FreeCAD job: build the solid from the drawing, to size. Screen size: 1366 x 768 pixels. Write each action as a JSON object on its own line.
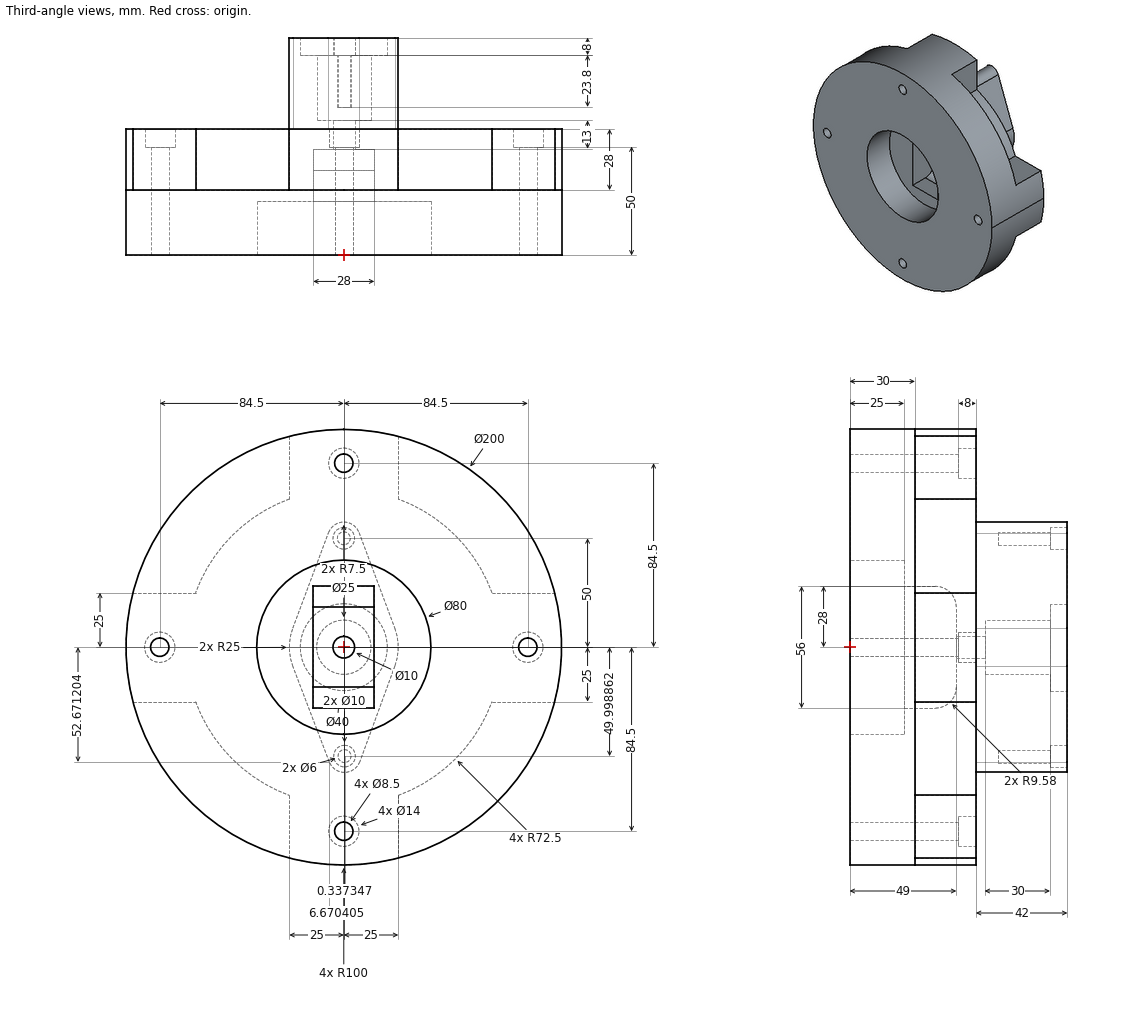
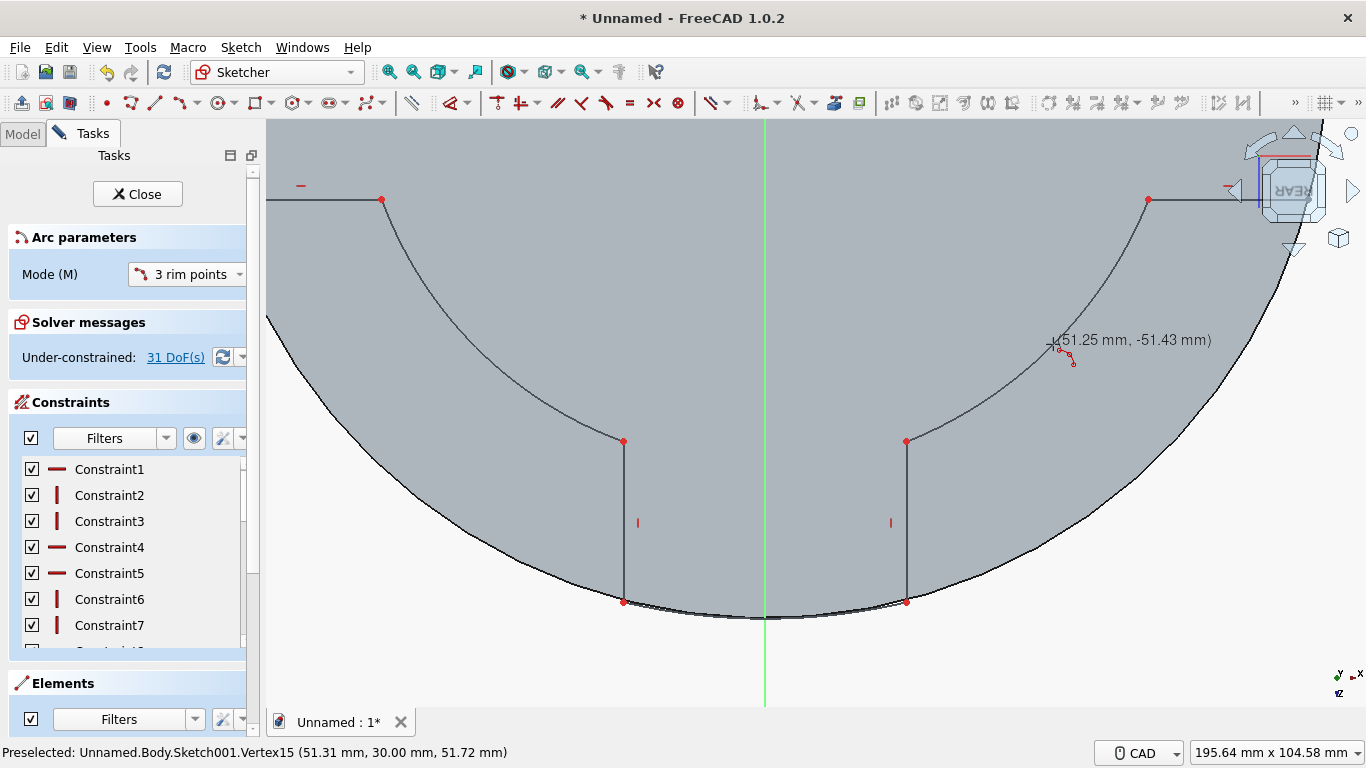
{"action": "scroll", "coordinate": [737, 621], "scroll_direction": "down", "scroll_amount": 5}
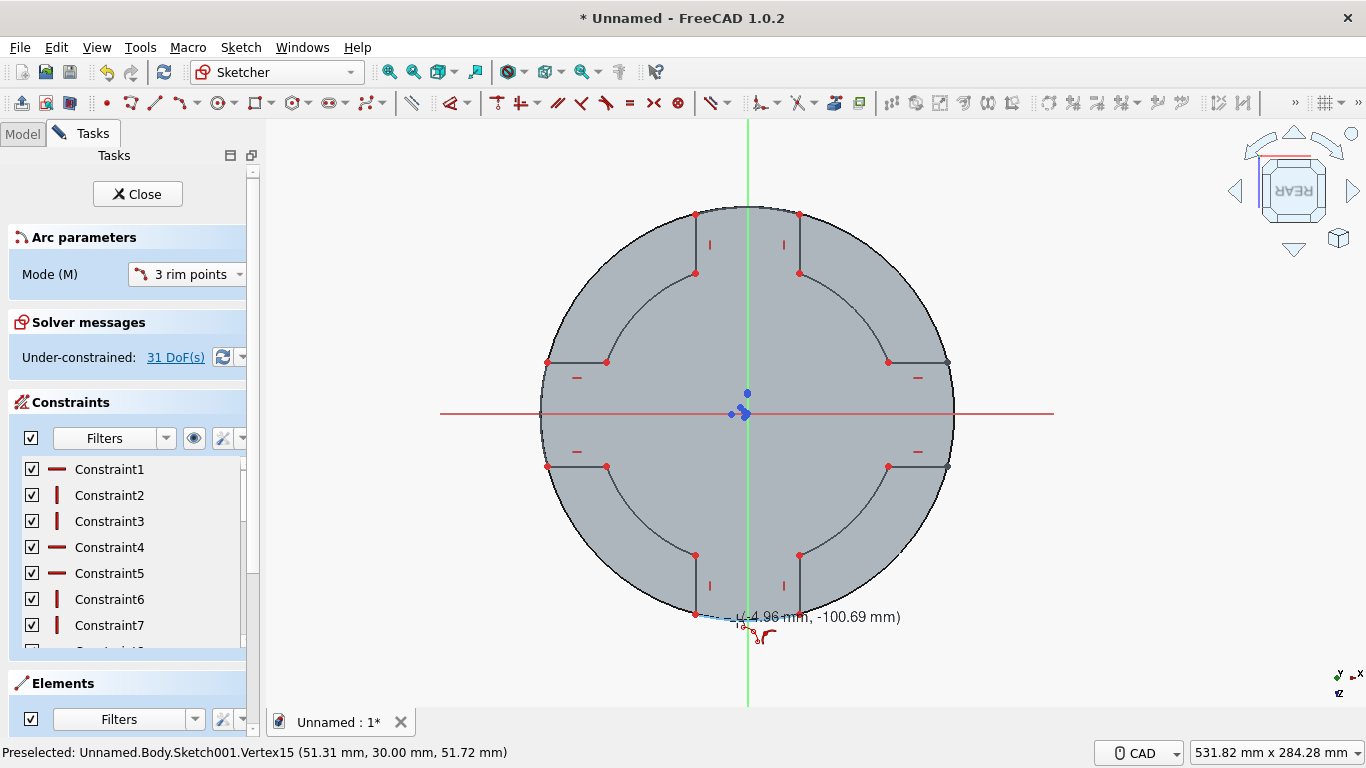
{"action": "left_click", "coordinate": [948, 467]}
{"action": "left_click", "coordinate": [948, 363]}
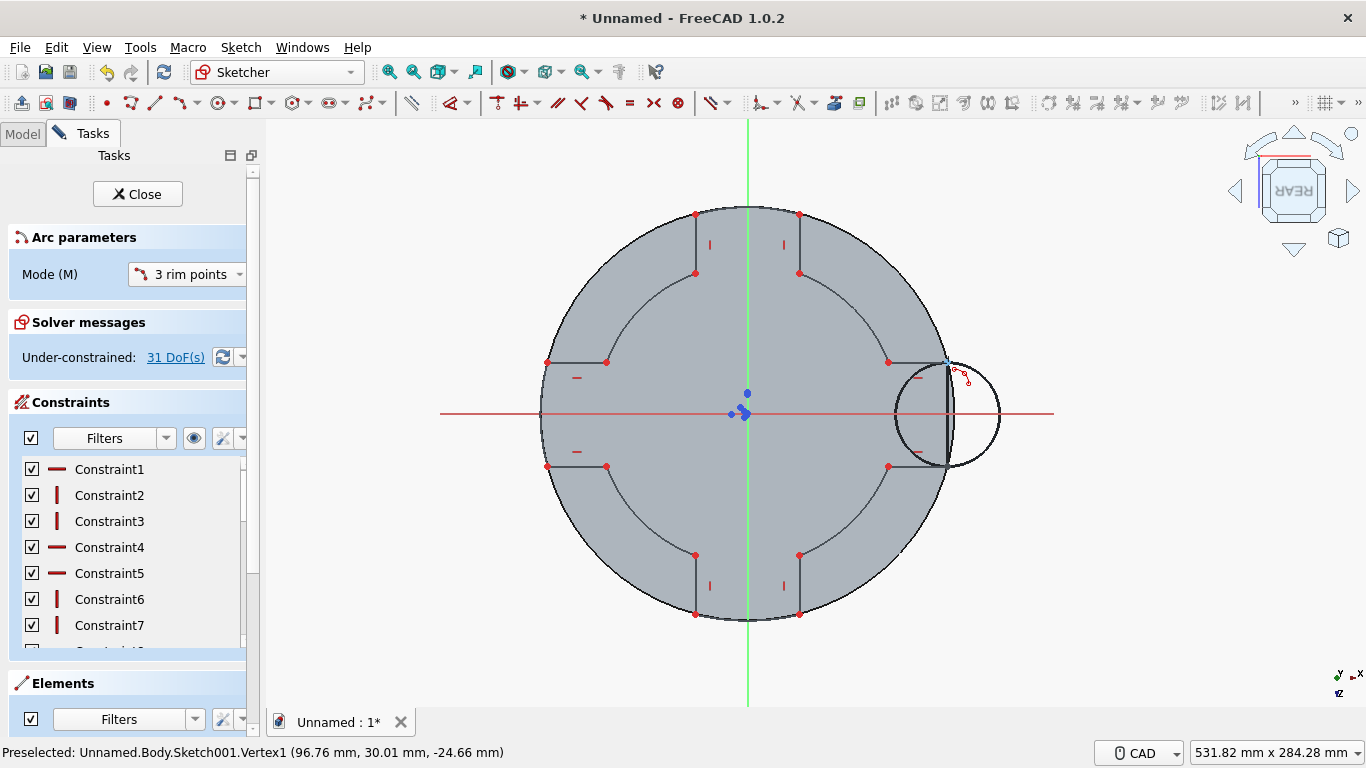
{"action": "scroll", "coordinate": [954, 424], "scroll_direction": "up", "scroll_amount": 5}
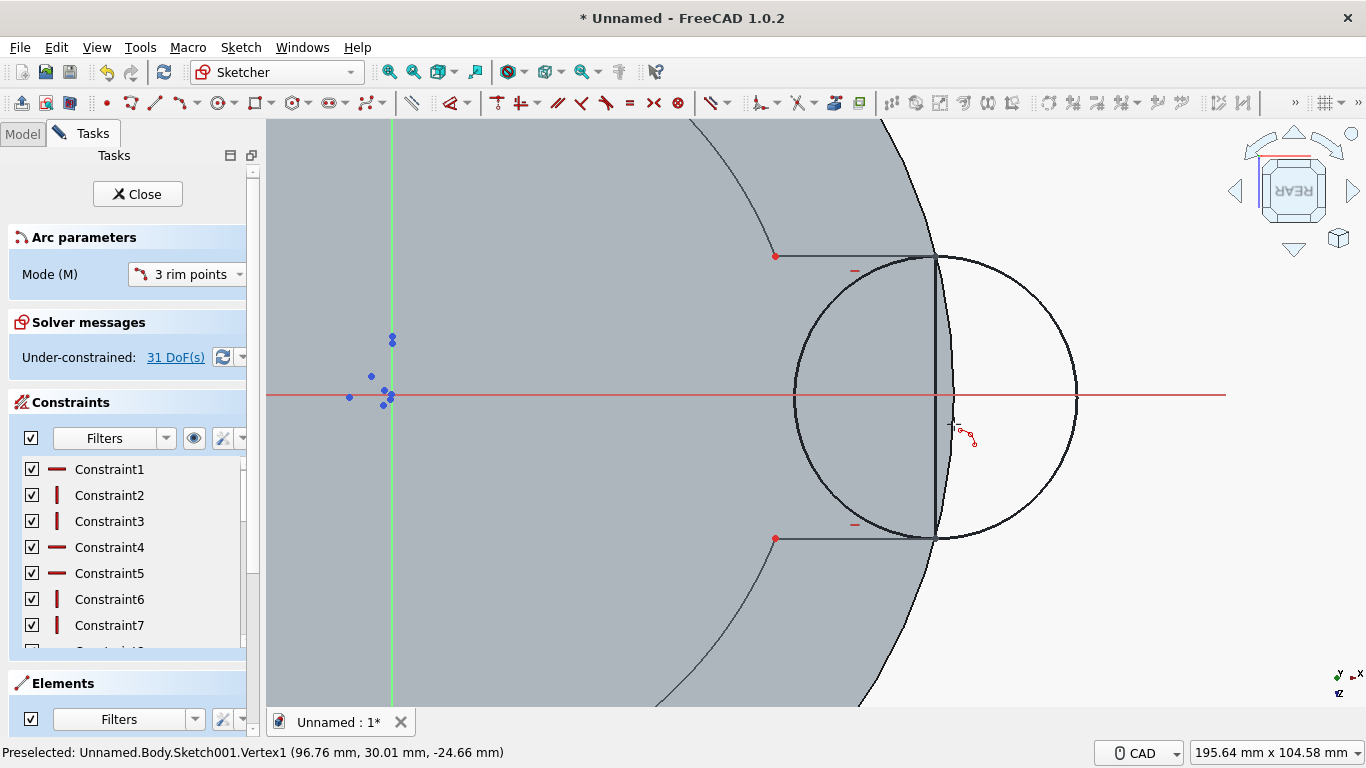
{"action": "left_click", "coordinate": [953, 423]}
{"action": "key", "text": "Escape"}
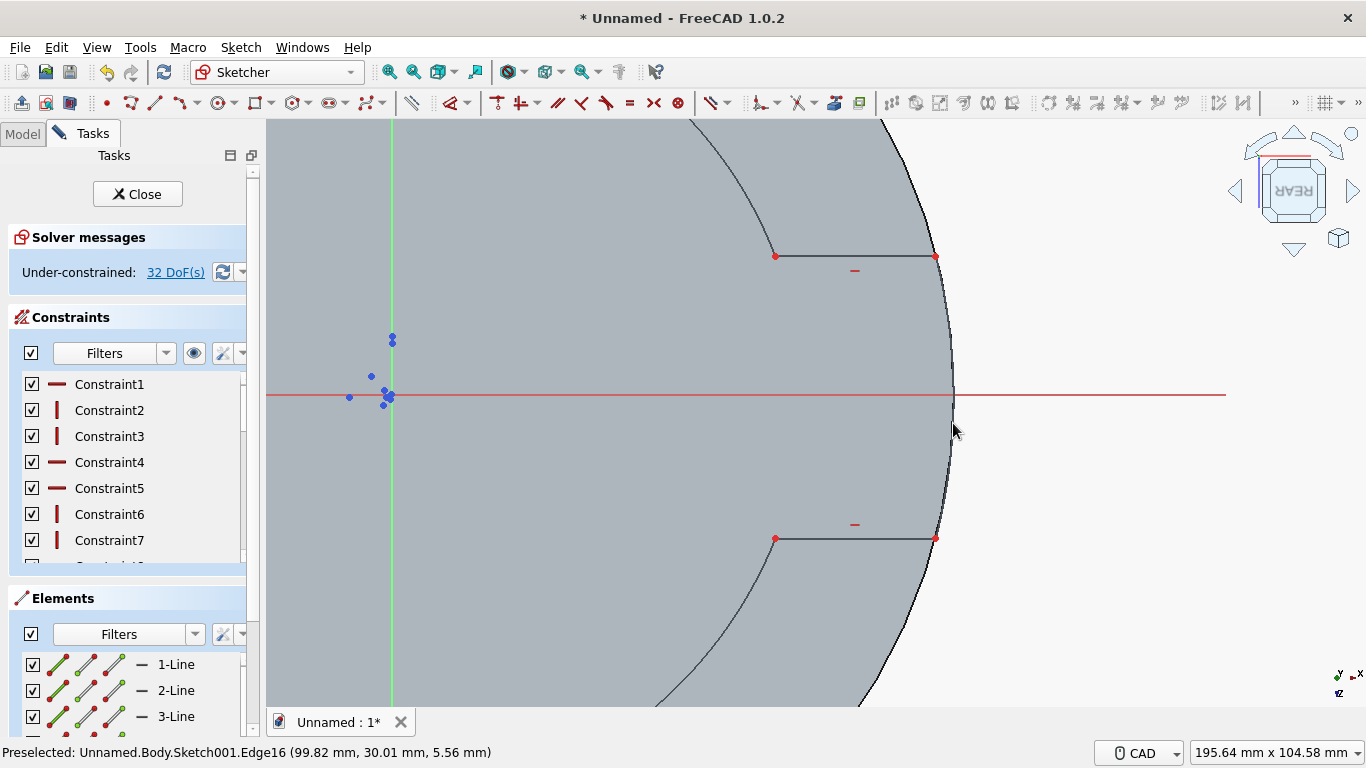
{"action": "left_click", "coordinate": [726, 163]}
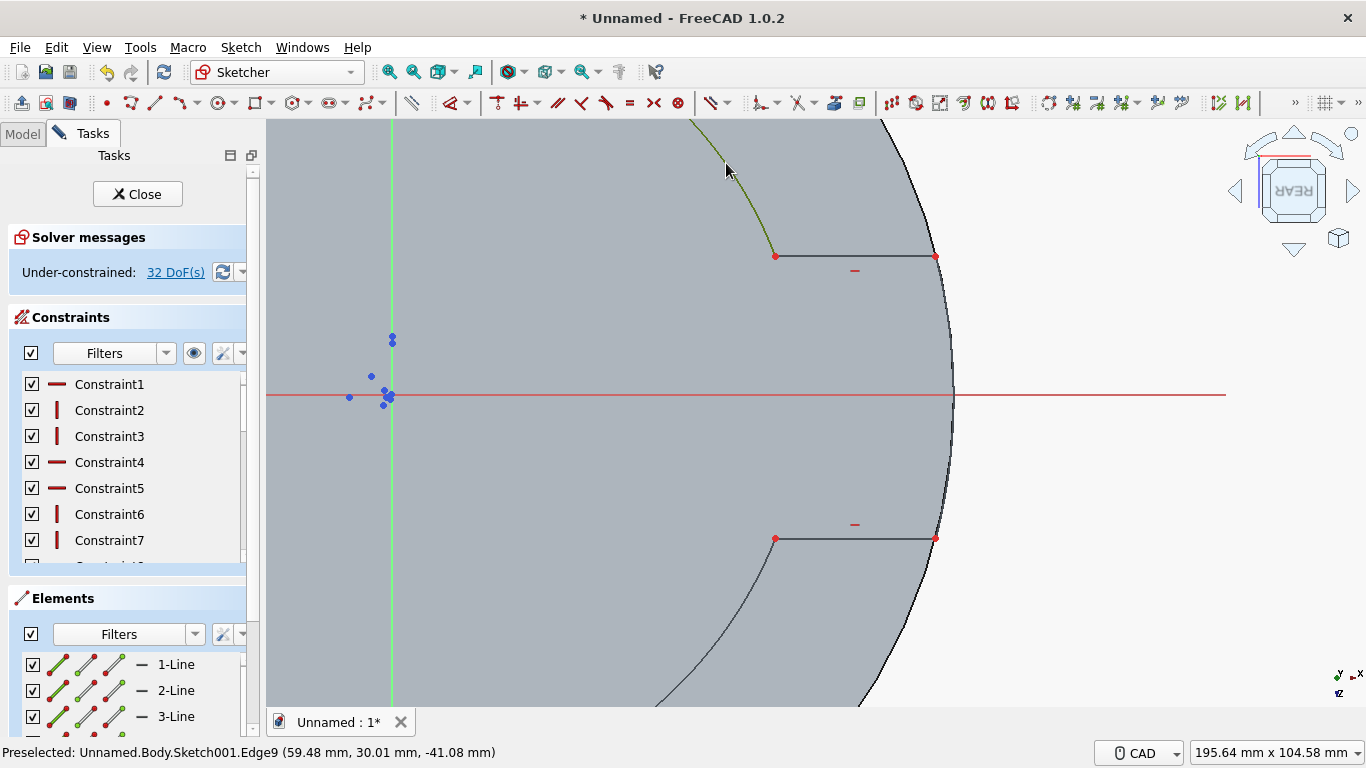
{"action": "scroll", "coordinate": [955, 424], "scroll_direction": "down", "scroll_amount": 5}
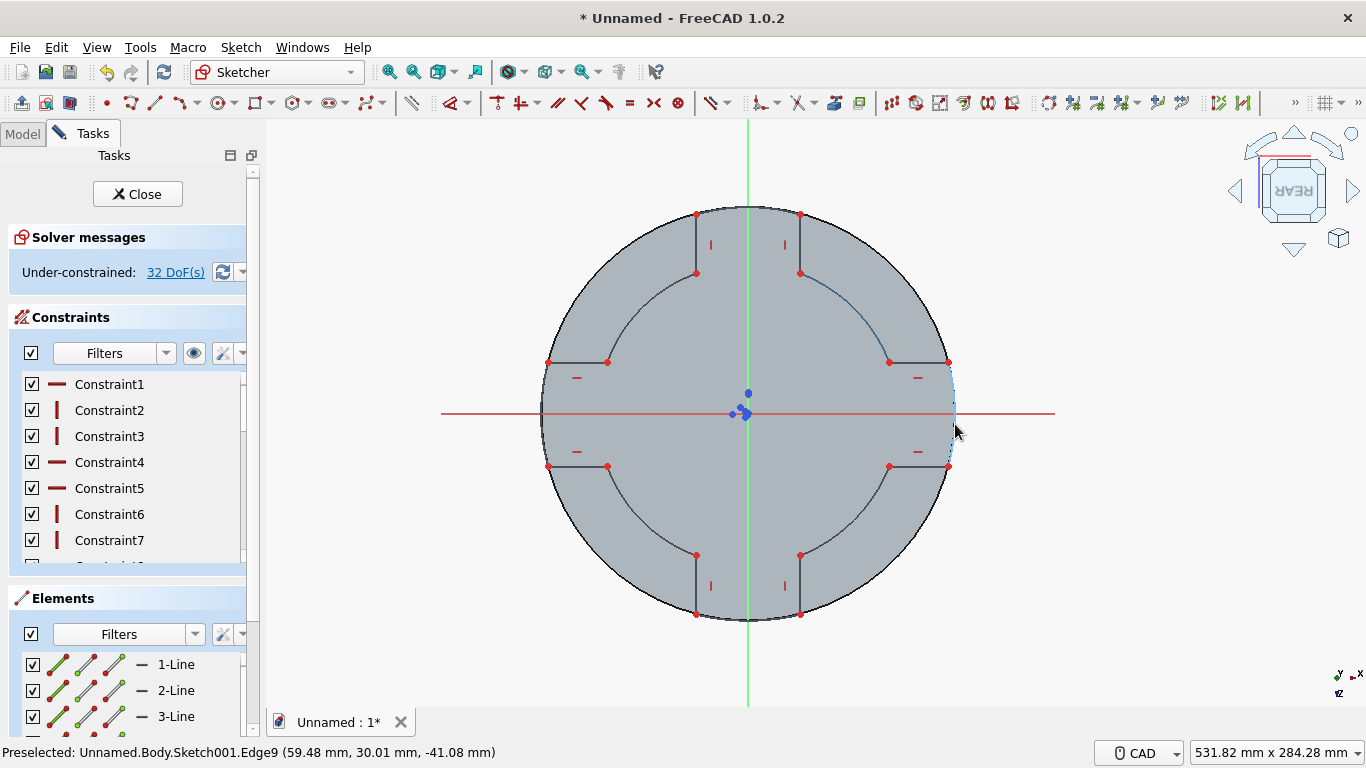
{"action": "left_click", "coordinate": [769, 208]}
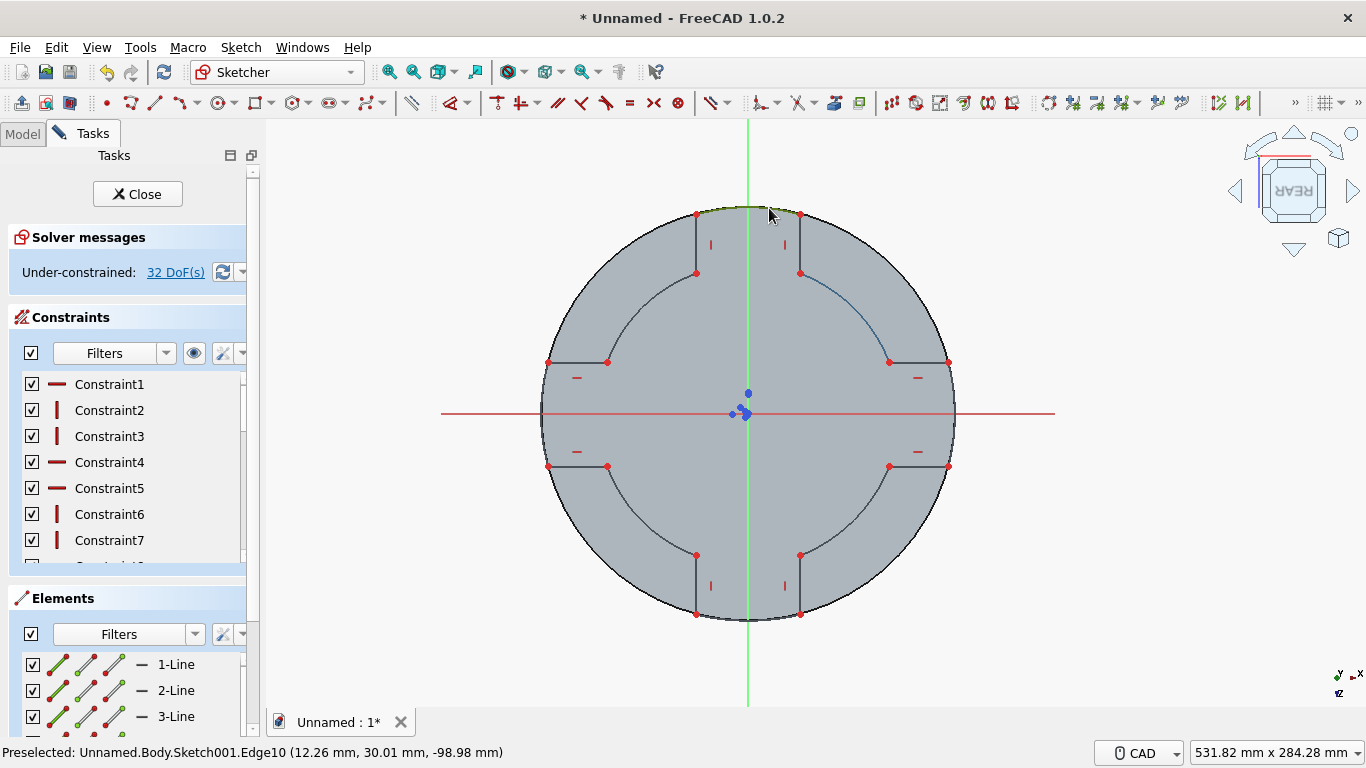
{"action": "key", "text": "c"}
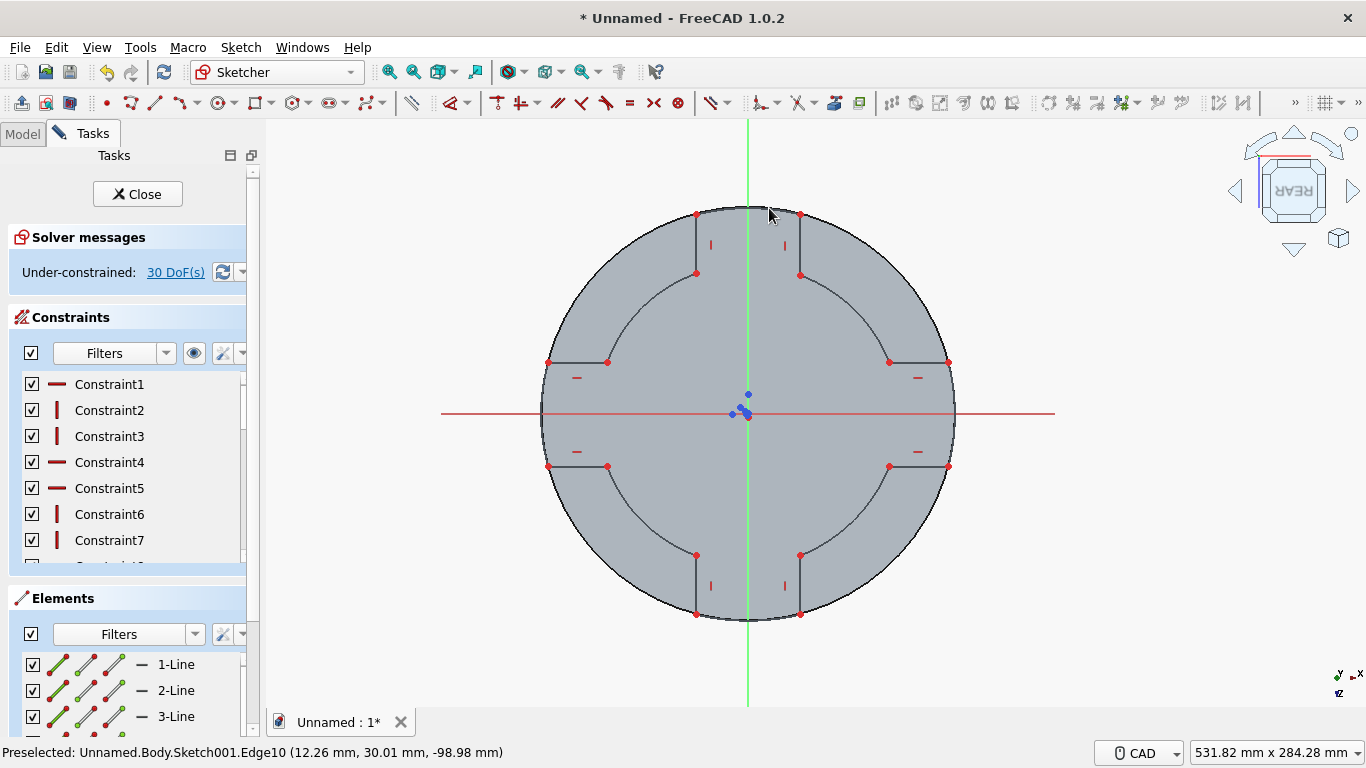
{"action": "left_click", "coordinate": [871, 329]}